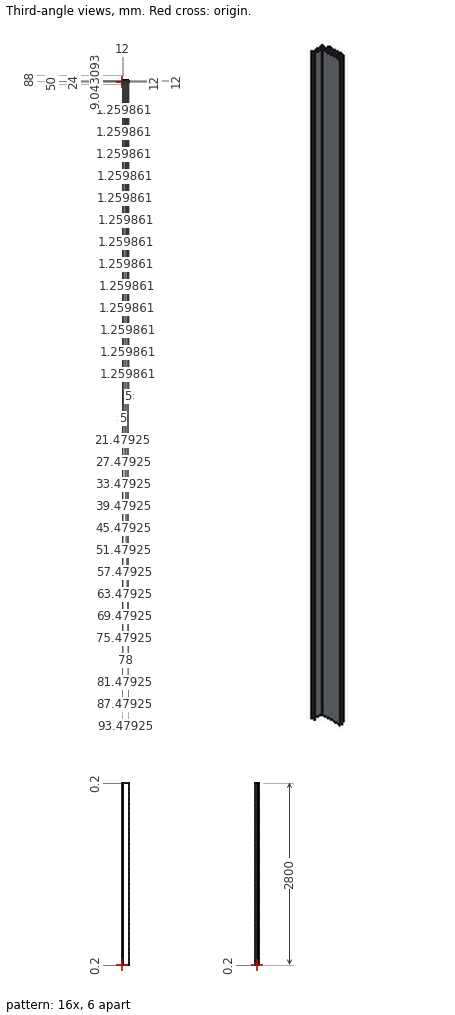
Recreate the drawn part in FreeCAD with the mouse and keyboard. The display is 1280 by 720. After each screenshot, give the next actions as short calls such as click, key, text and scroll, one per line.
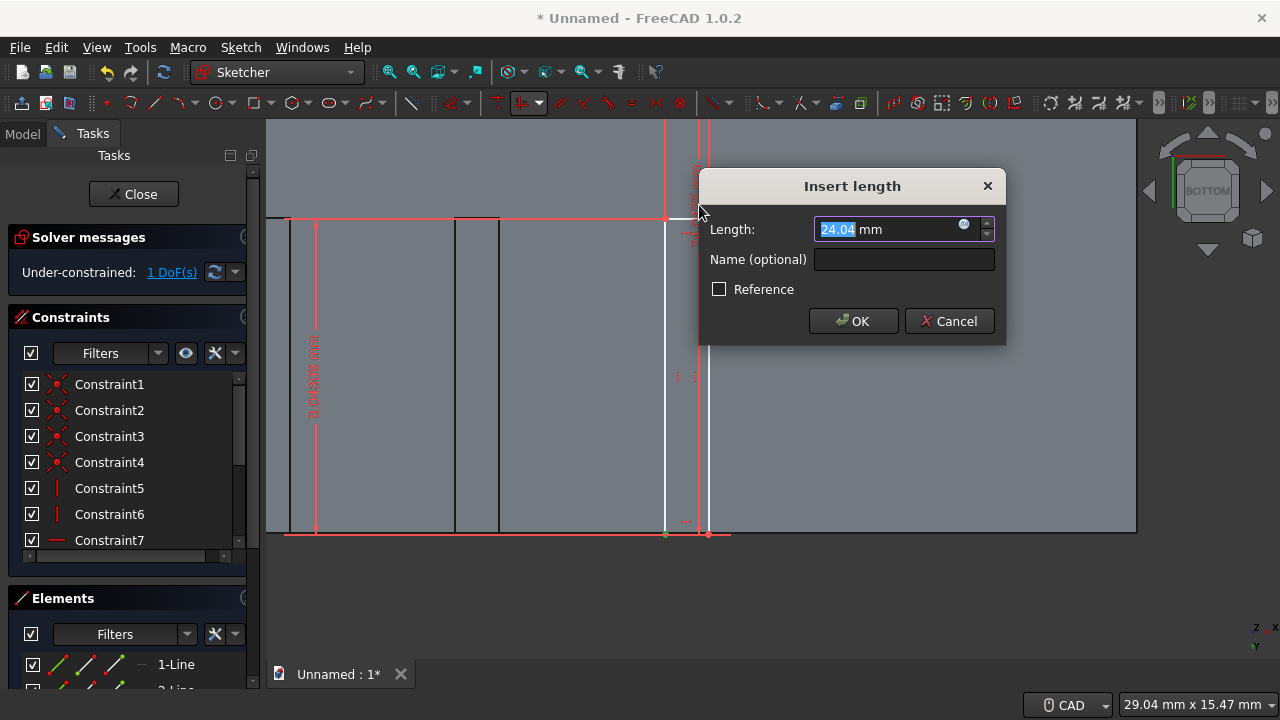
text(24)
key(Return)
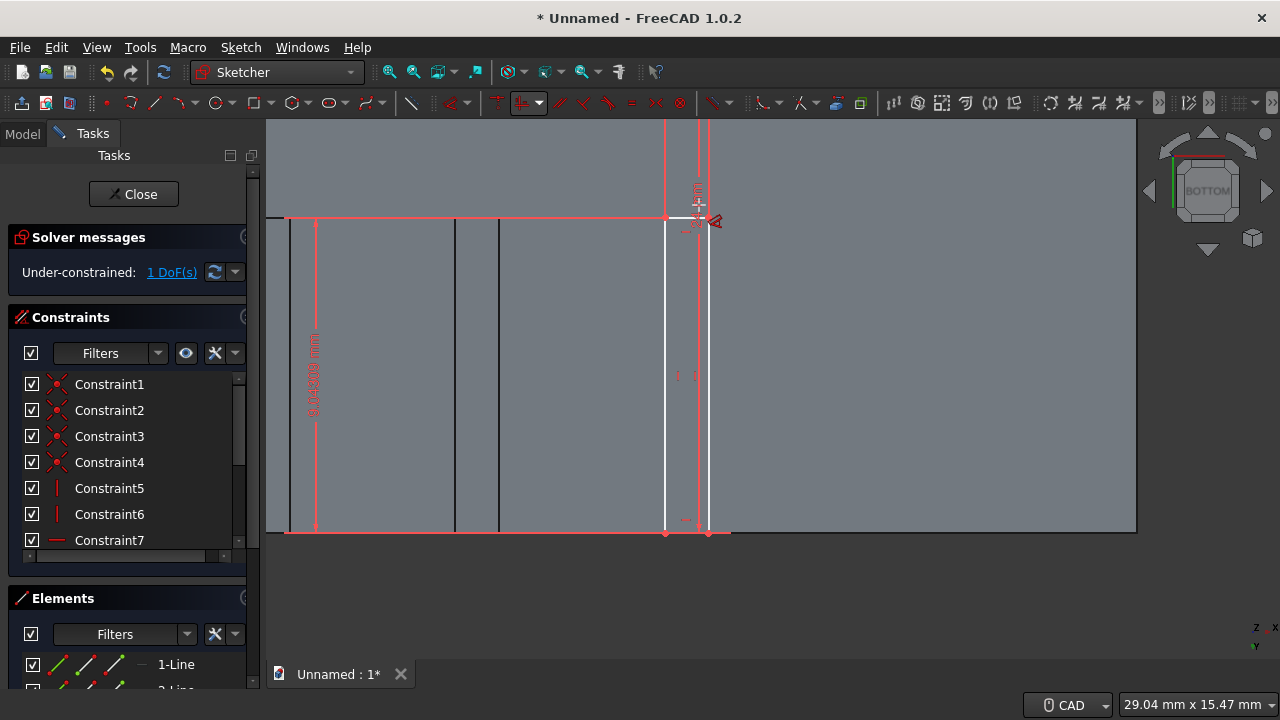
click(665, 218)
click(479, 252)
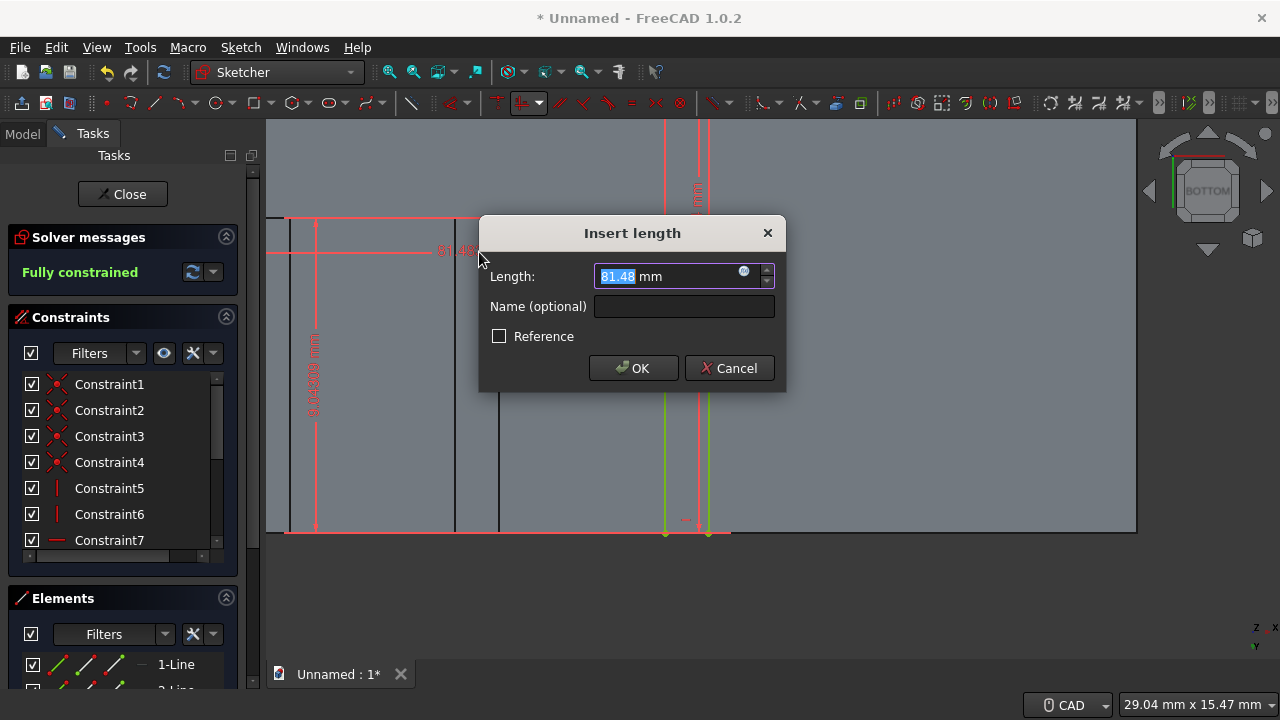
text(81.47925)
key(Return)
key(Escape)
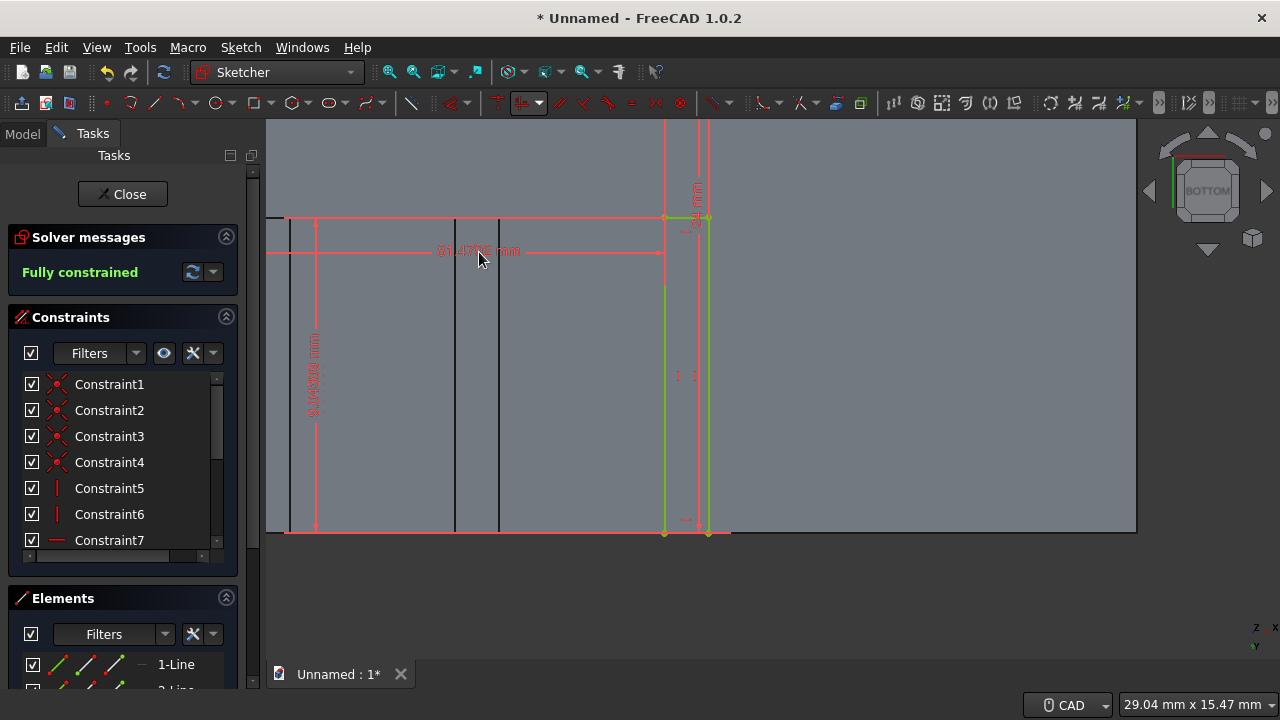
click(123, 194)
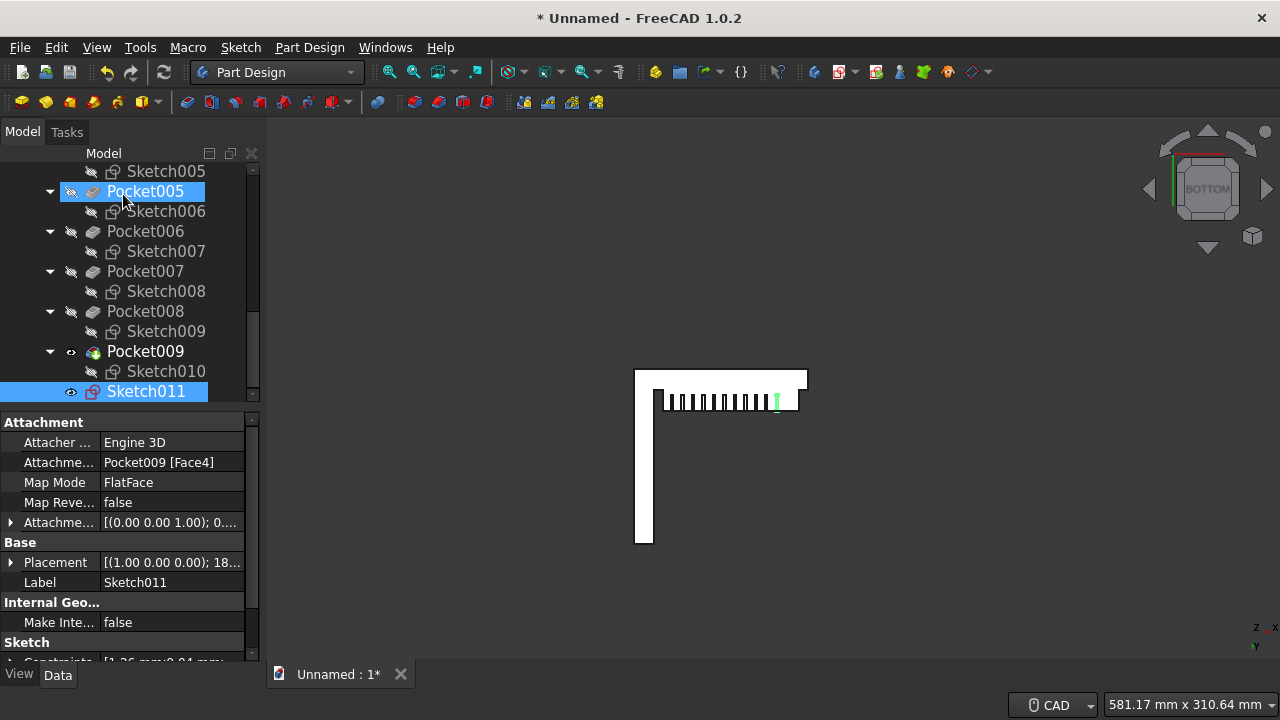
click(188, 102)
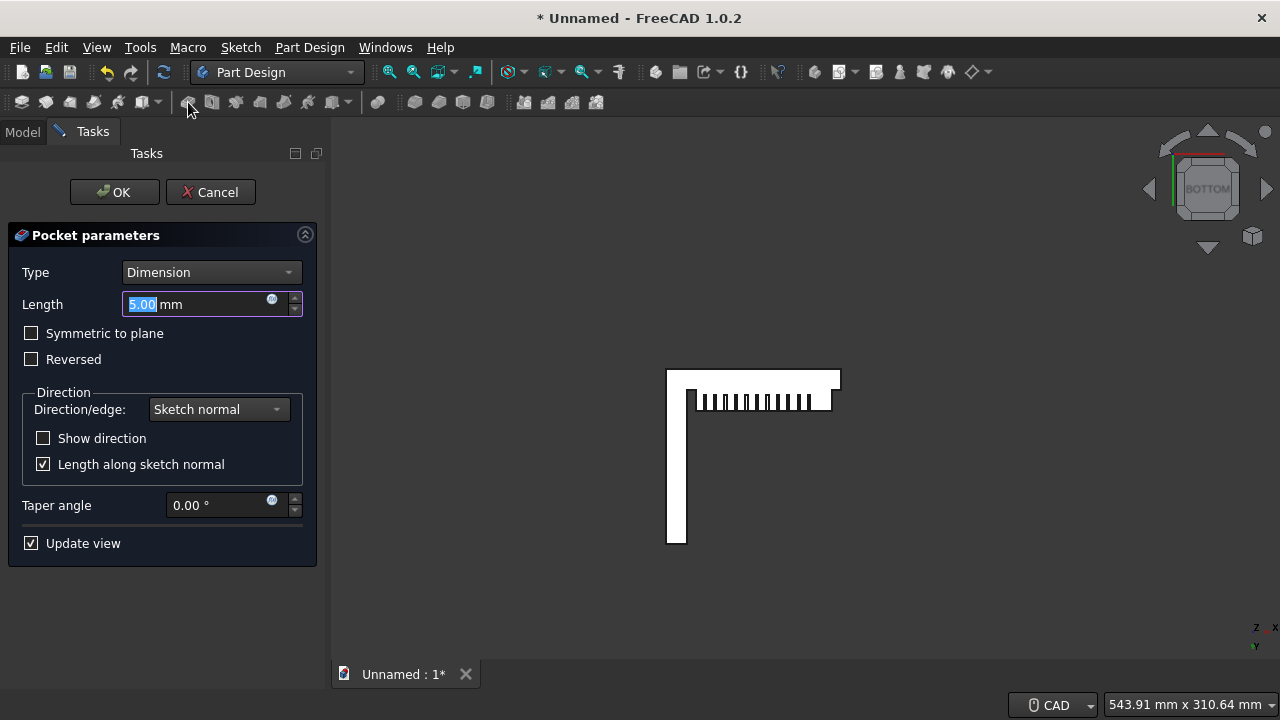
text(0.2)
key(Tab)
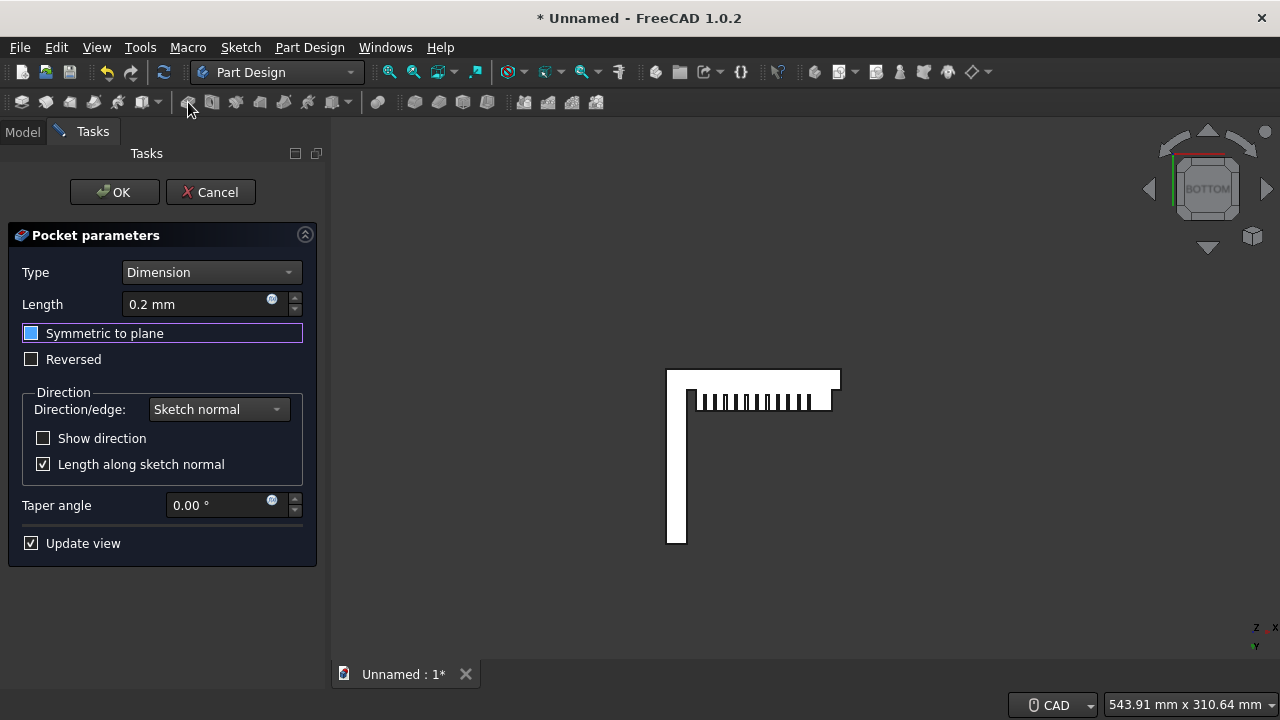
click(115, 192)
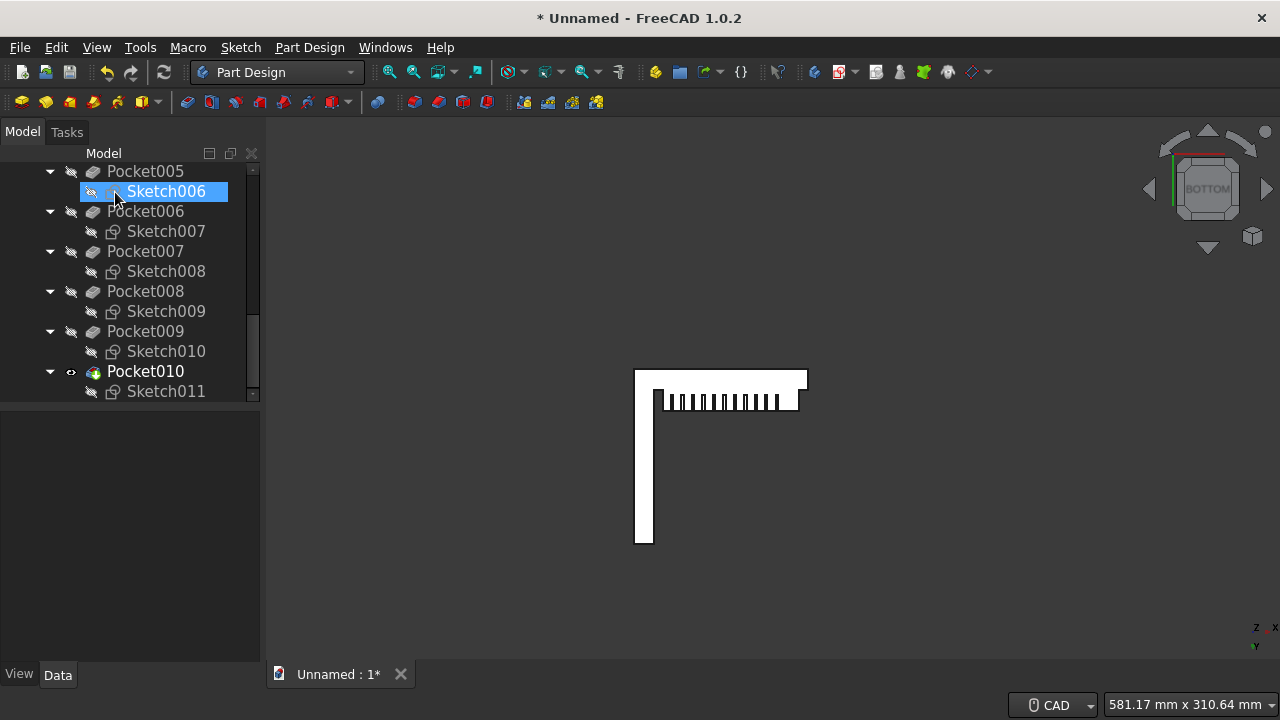
click(390, 72)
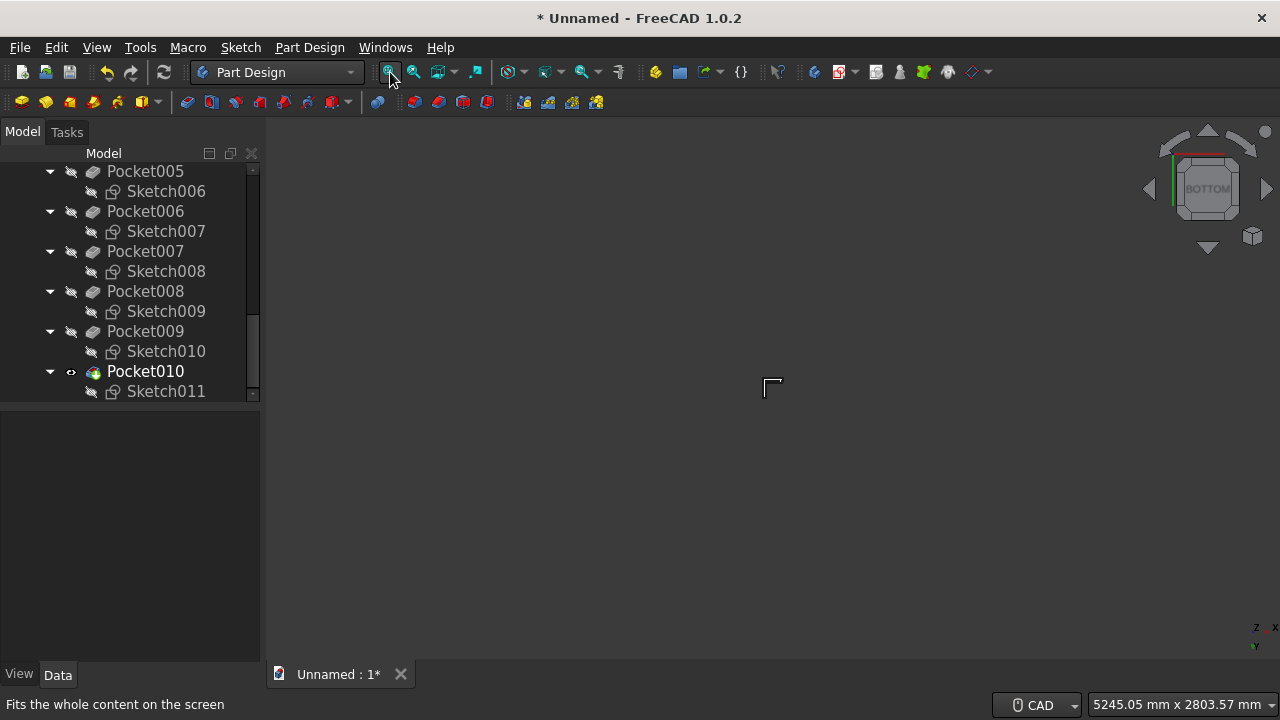
scroll(779, 379, up, 11)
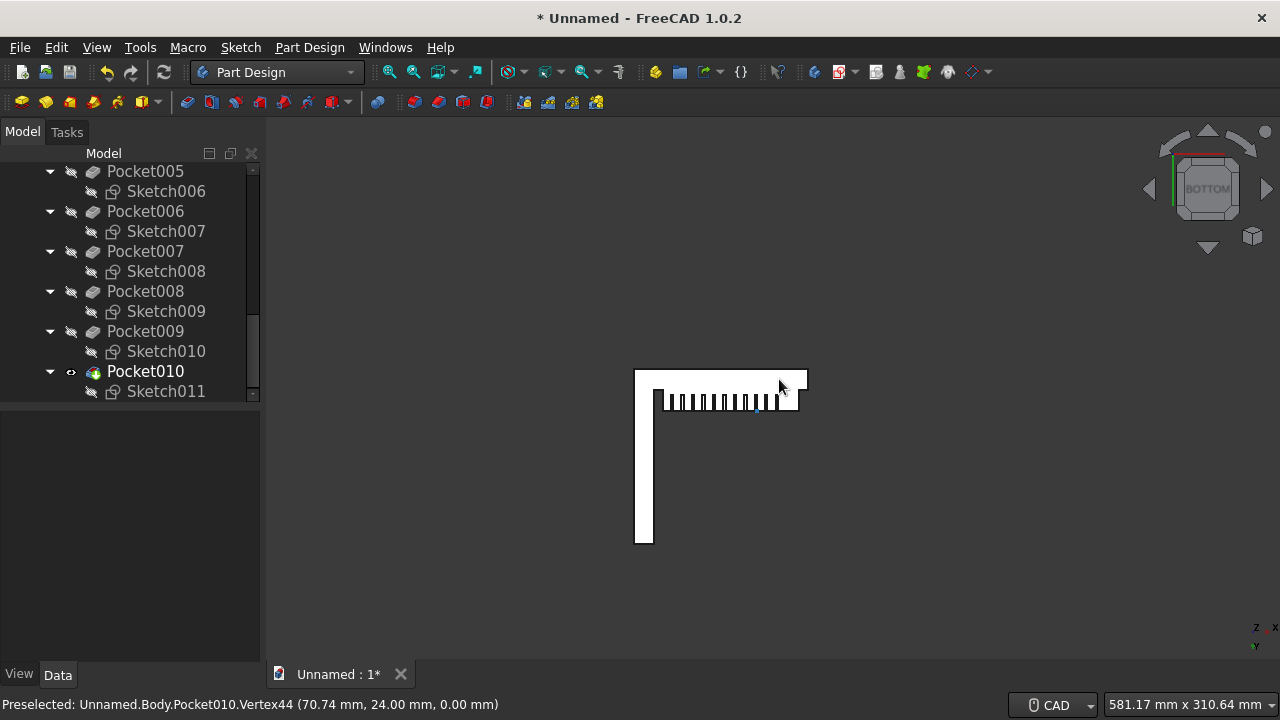
click(771, 381)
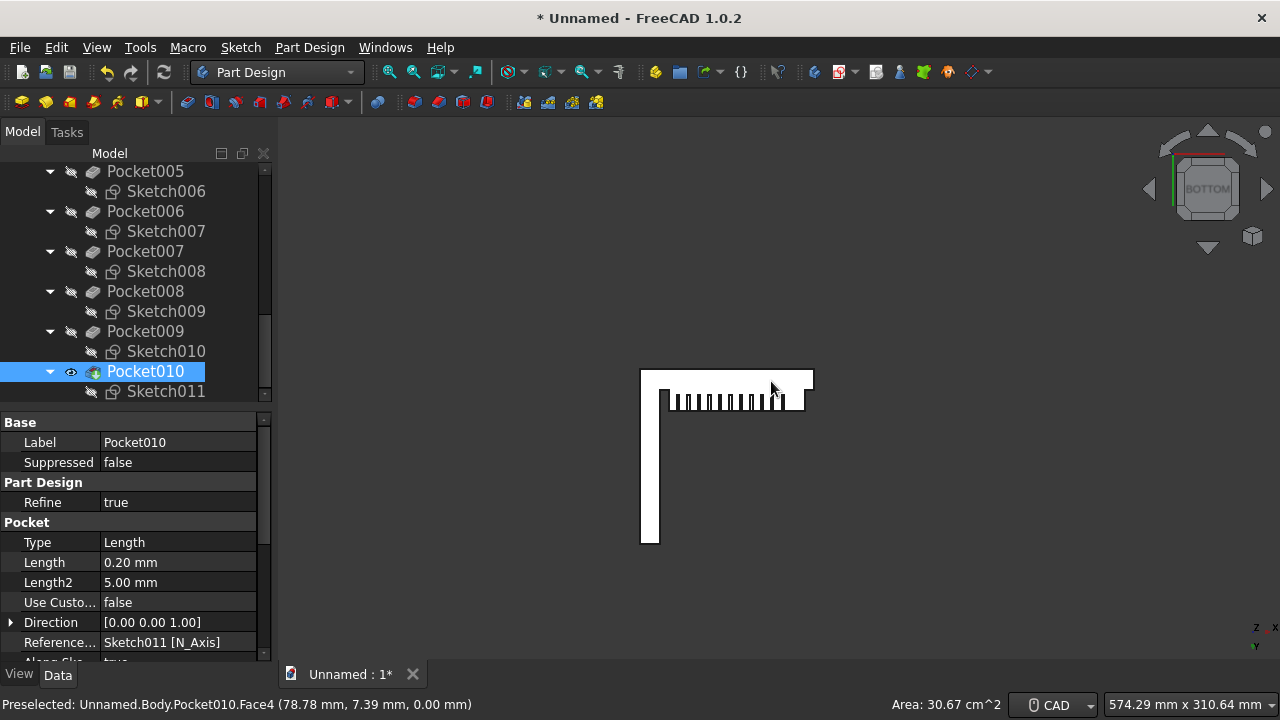
click(840, 72)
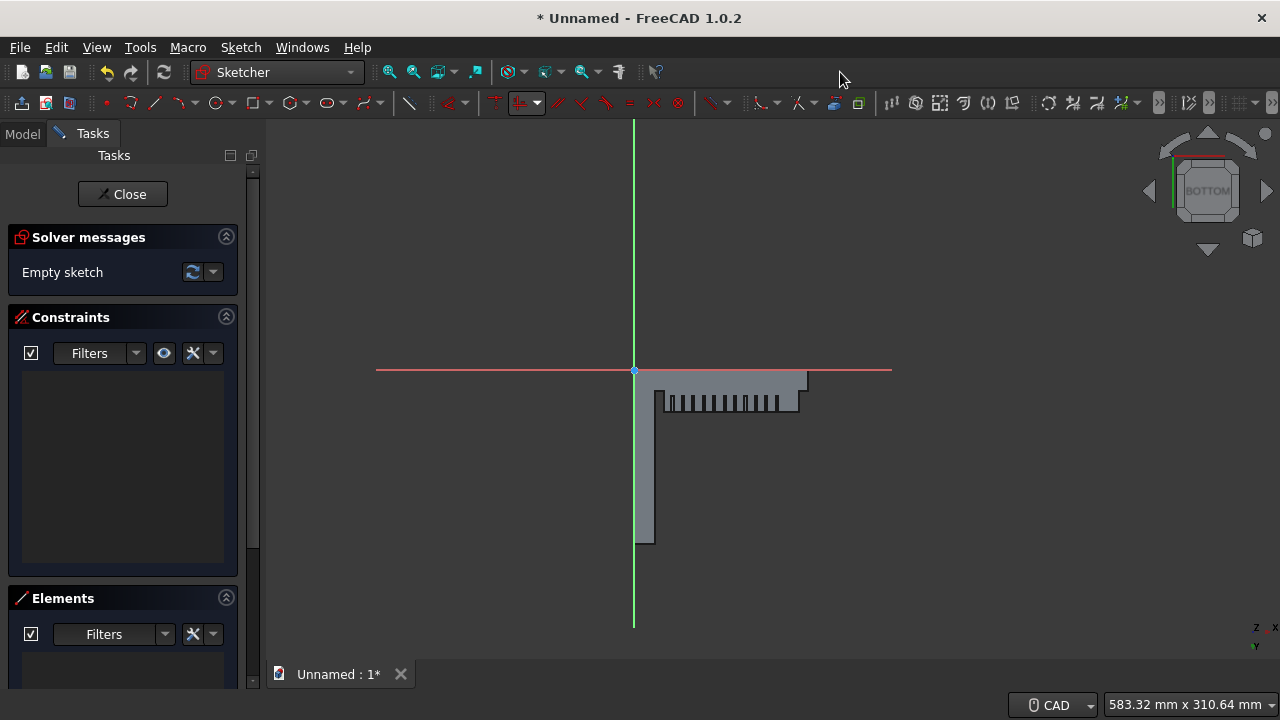
scroll(792, 405, up, 15)